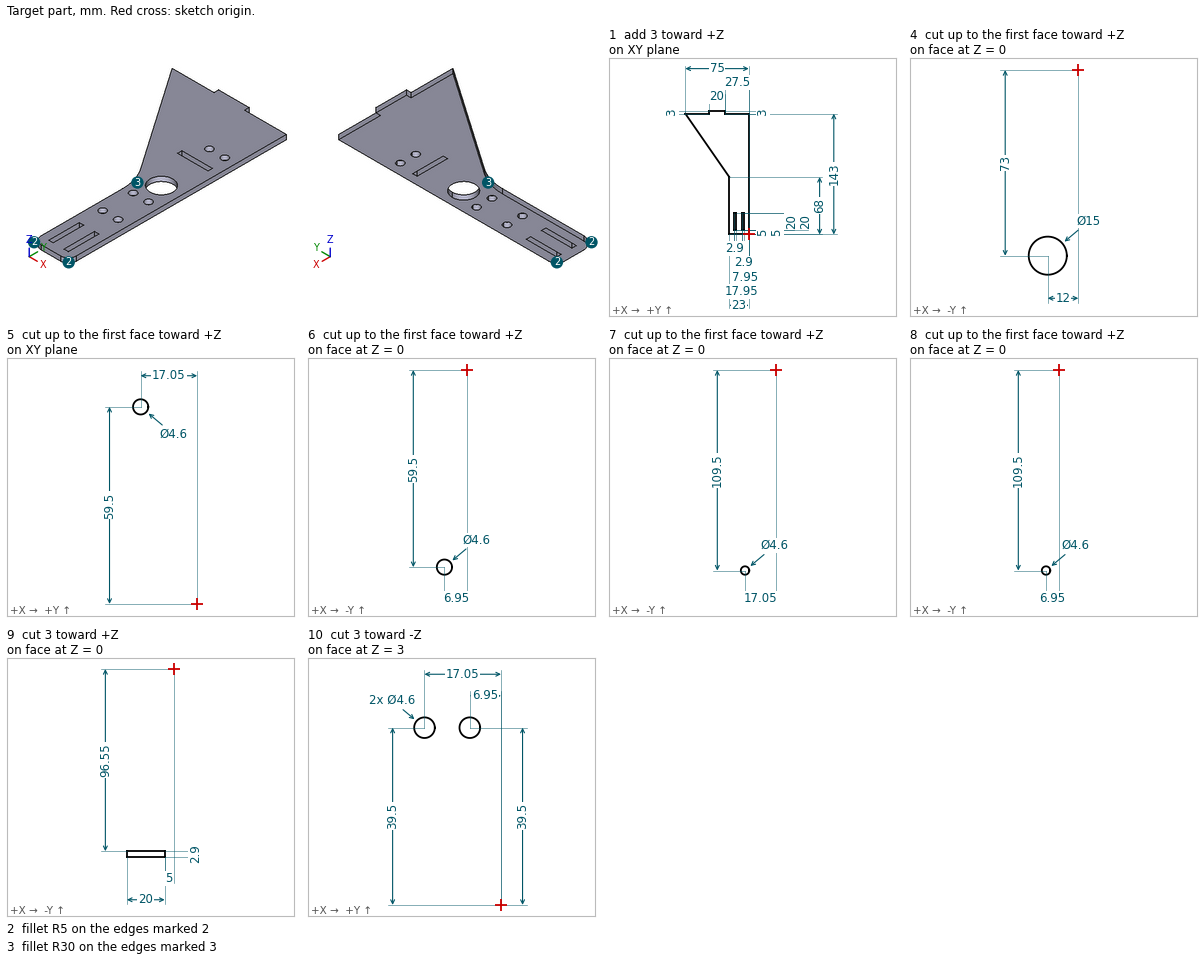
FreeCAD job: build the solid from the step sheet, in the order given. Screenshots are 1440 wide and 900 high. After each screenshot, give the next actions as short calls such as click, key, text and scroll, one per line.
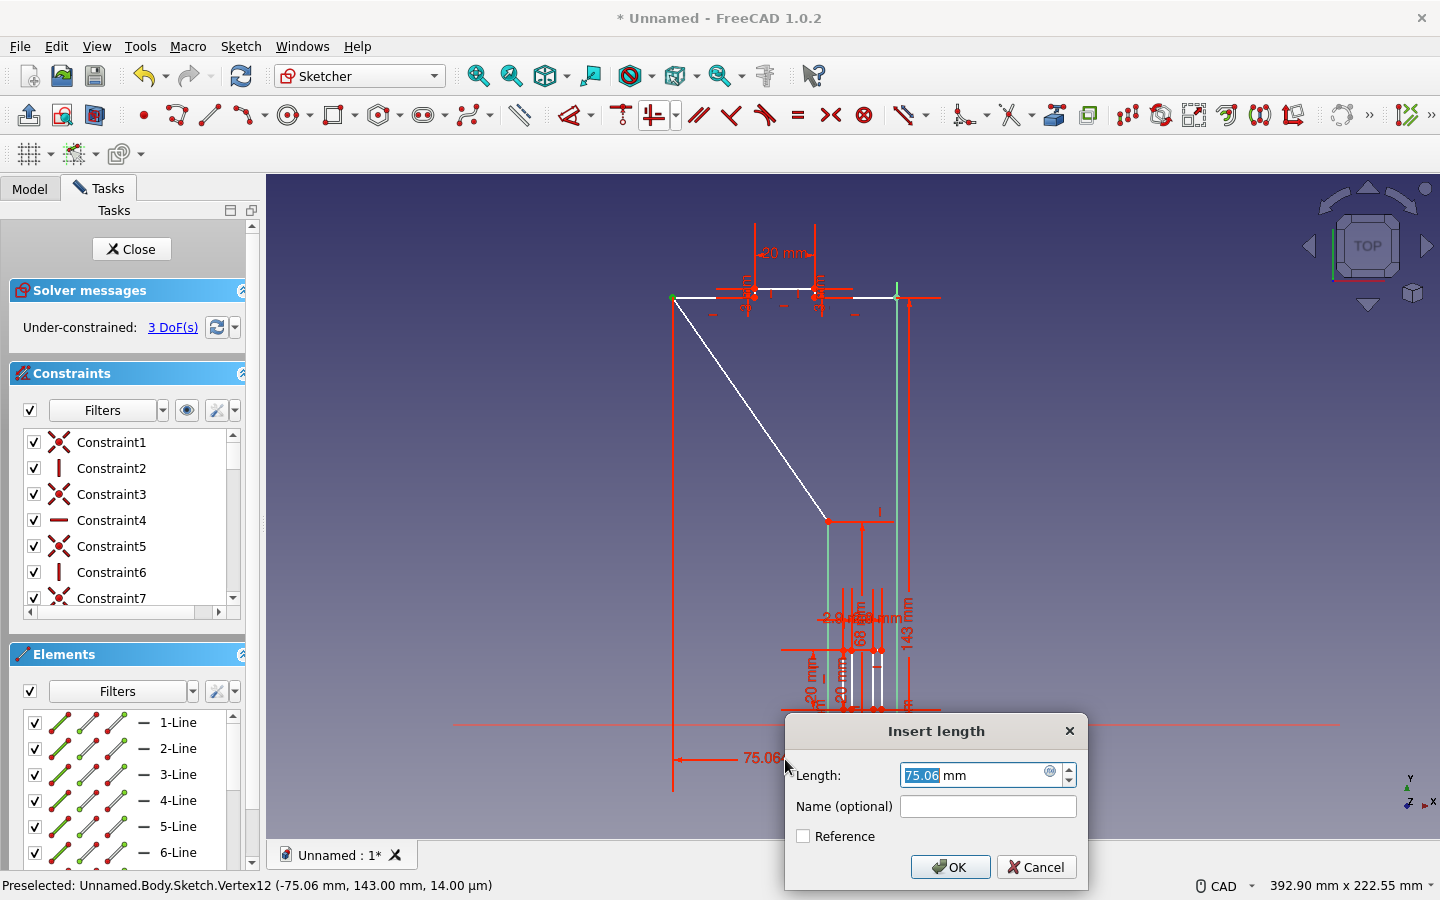
text(75)
key(Return)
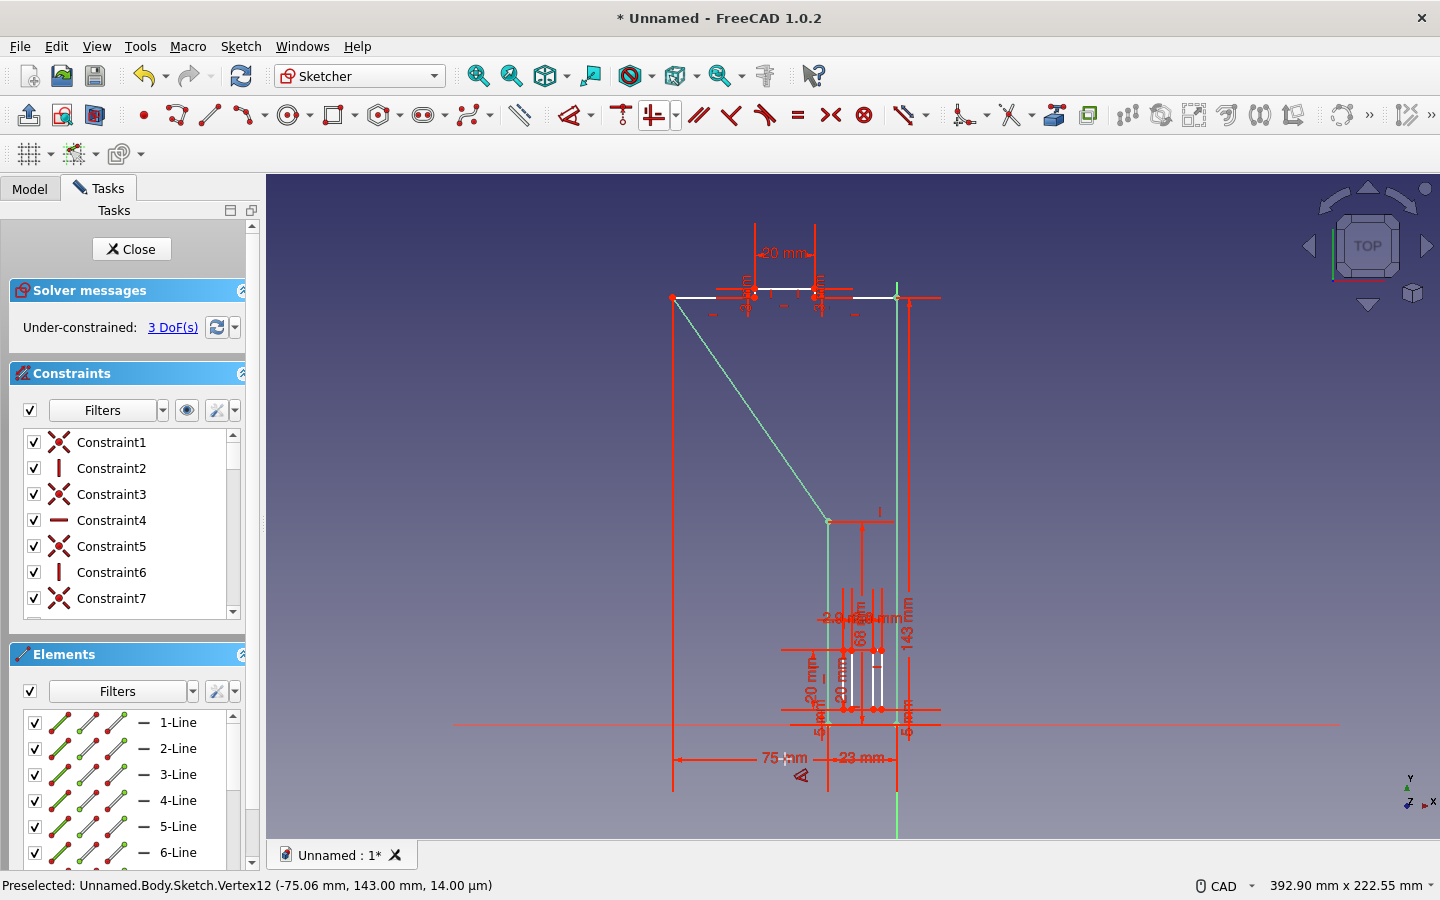
click(872, 298)
click(856, 264)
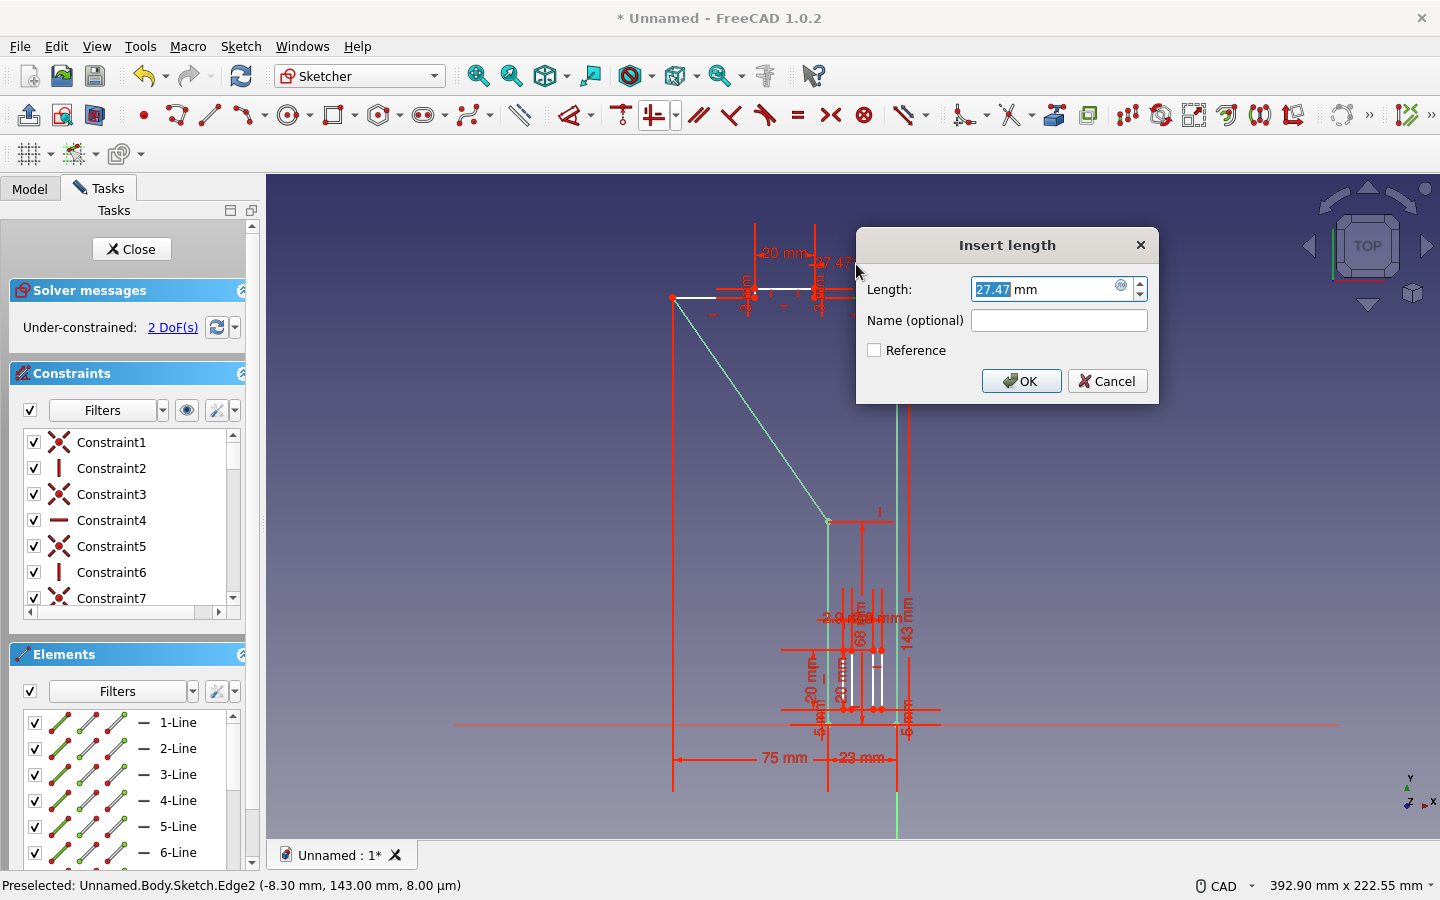
text(27.5)
key(Return)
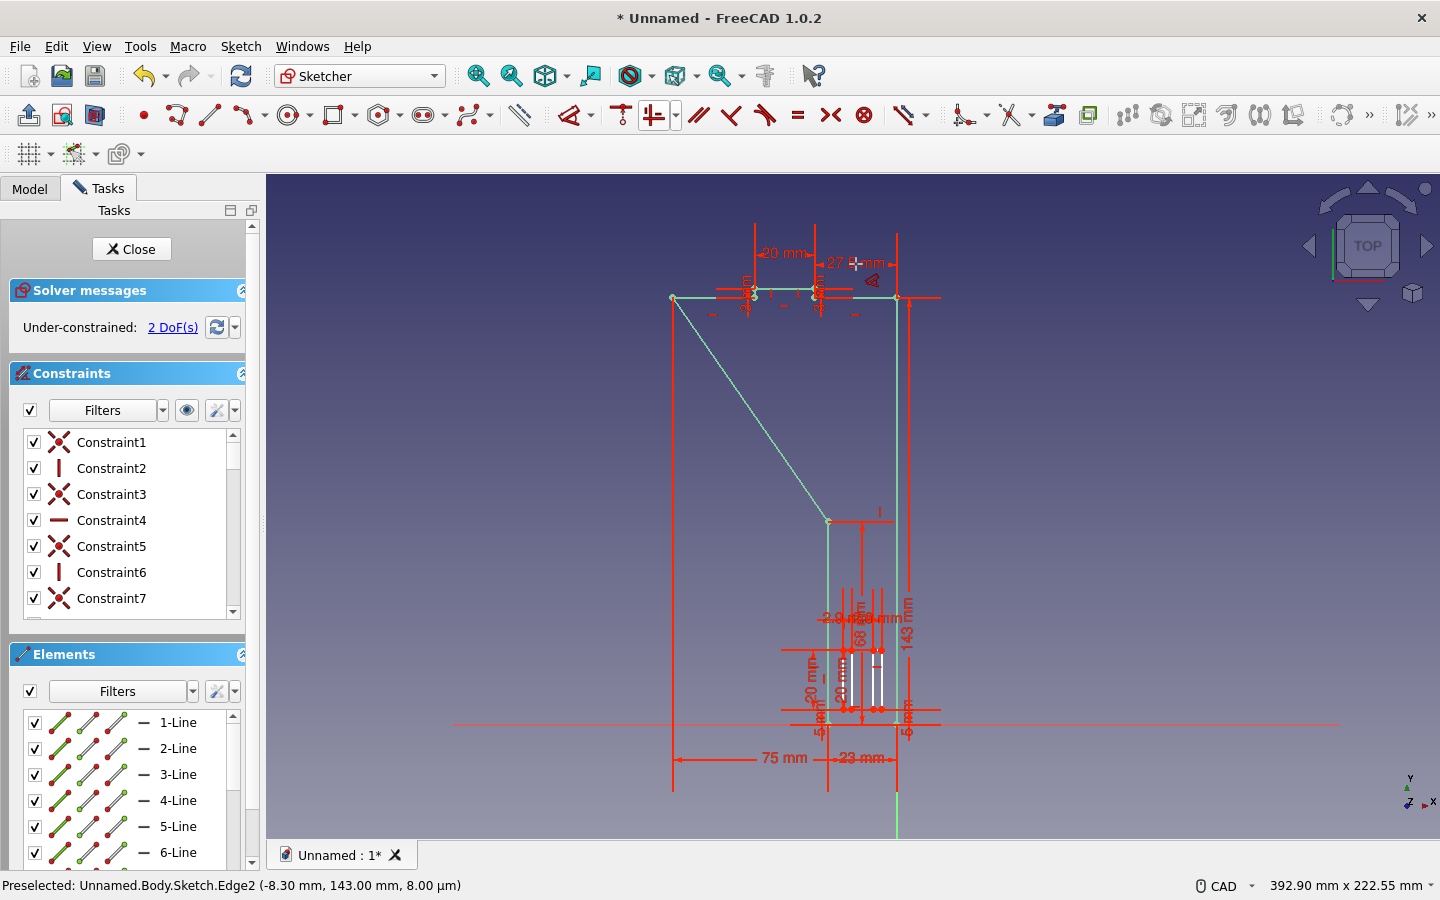
scroll(873, 650, up, 3)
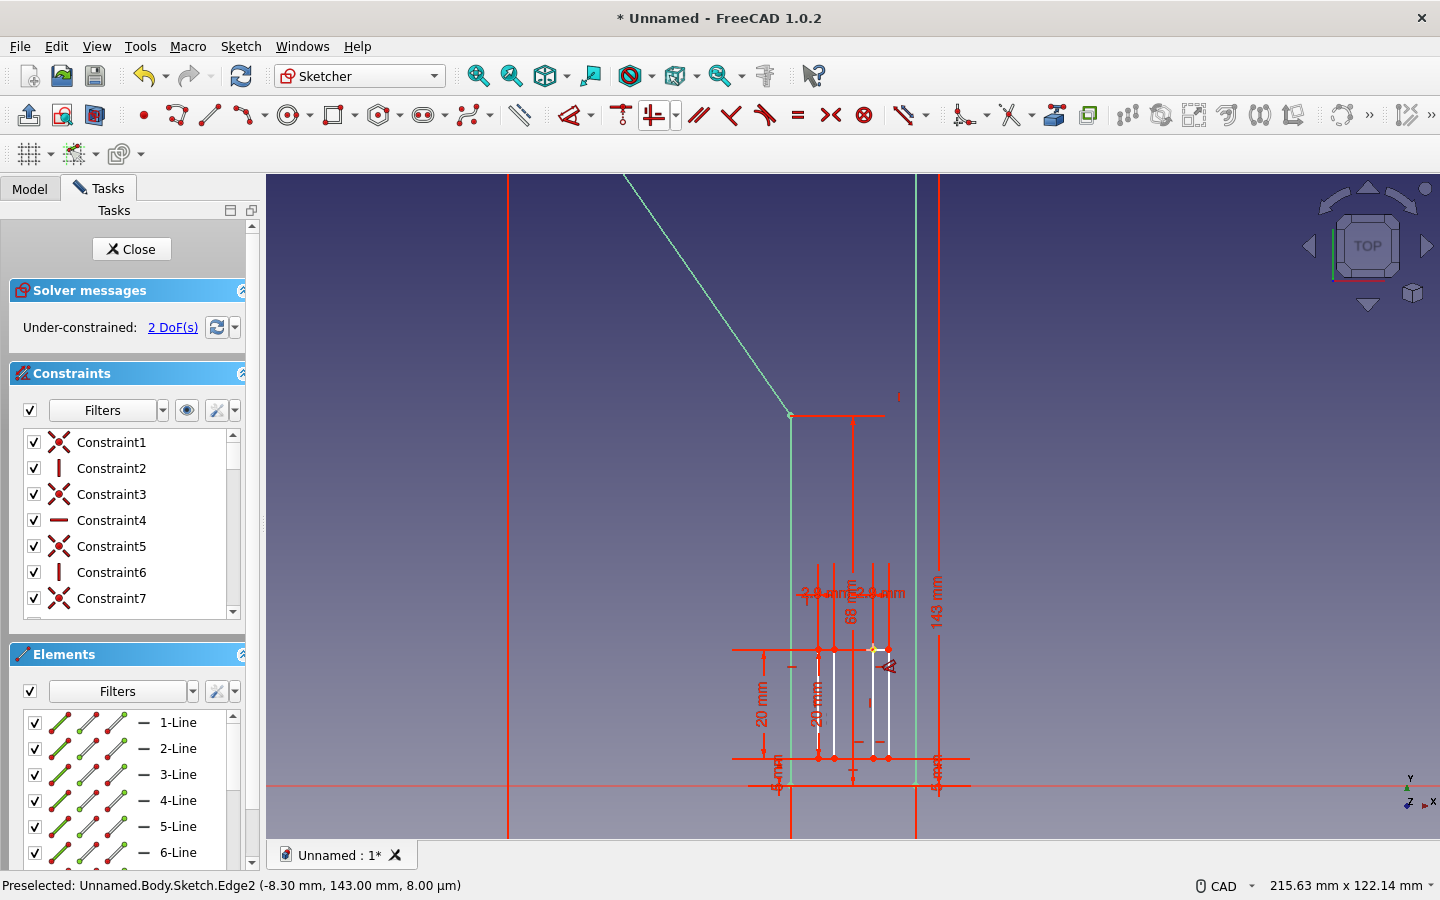
click(873, 650)
click(895, 568)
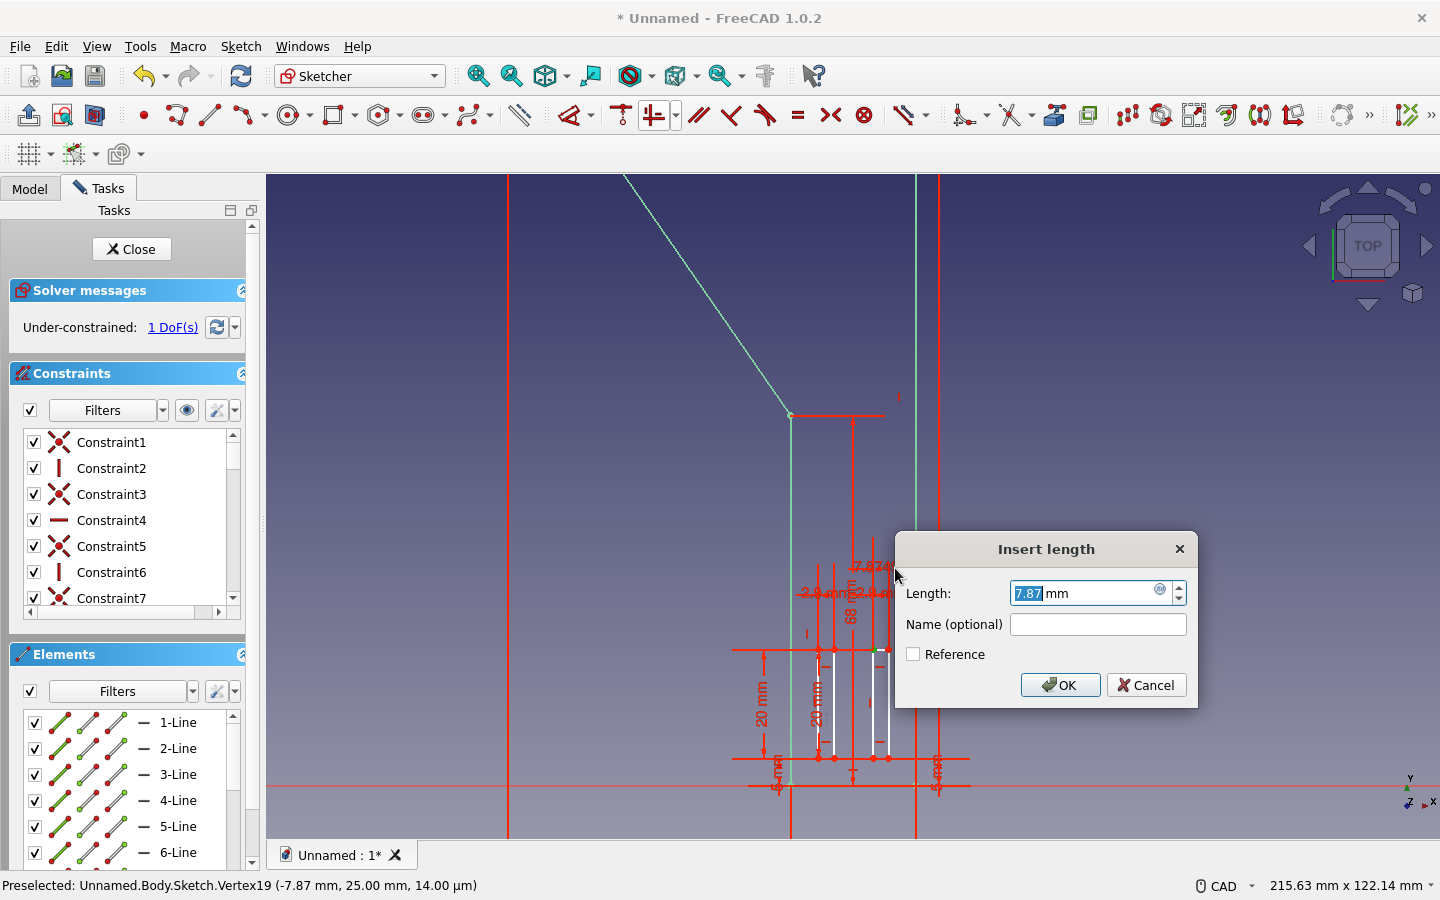
text(7.95)
key(Return)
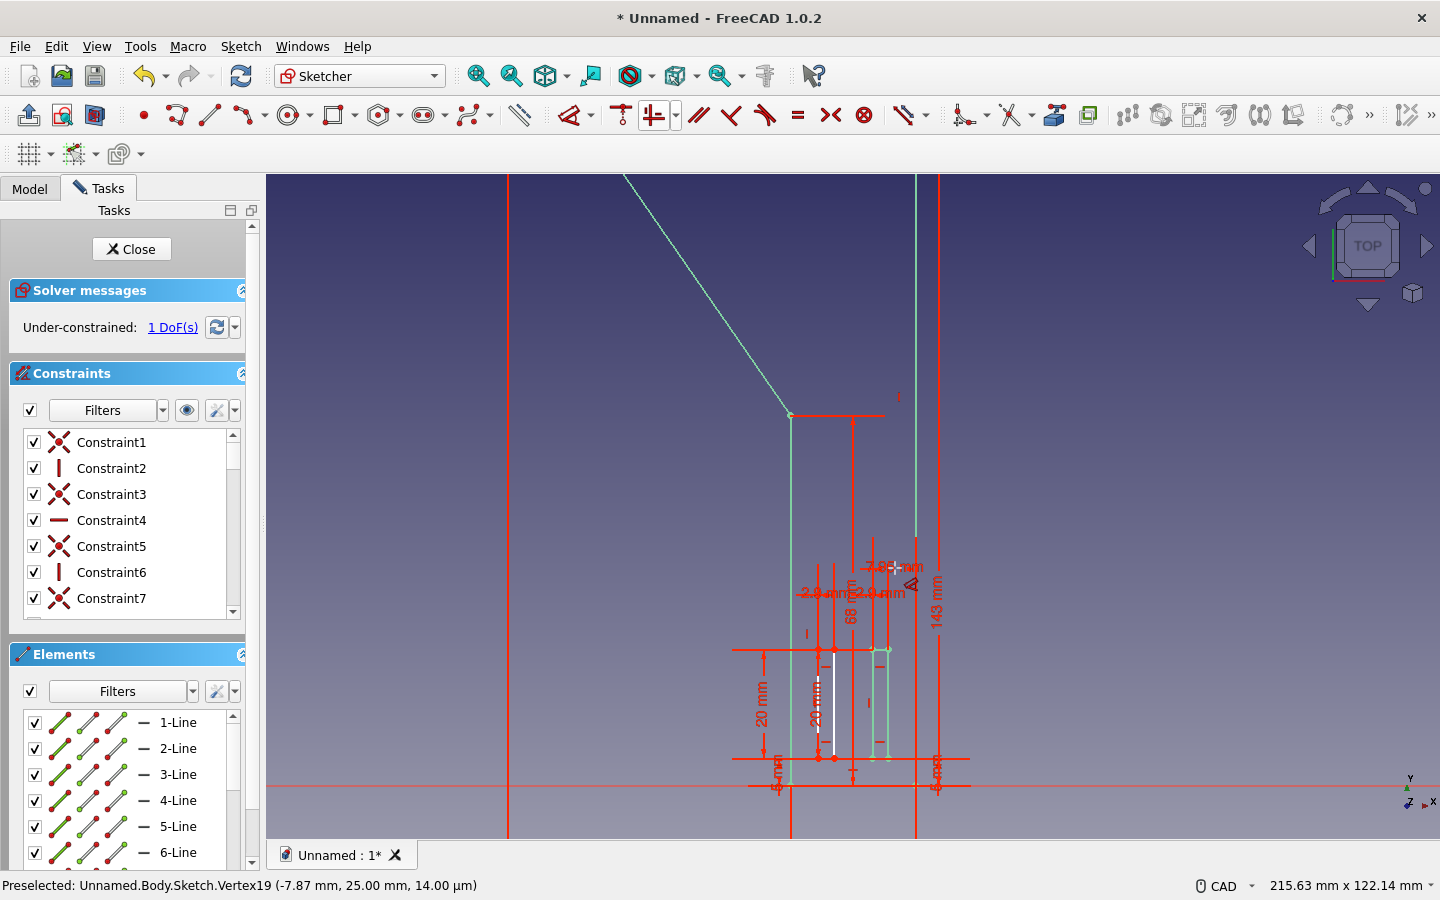
click(818, 650)
click(867, 544)